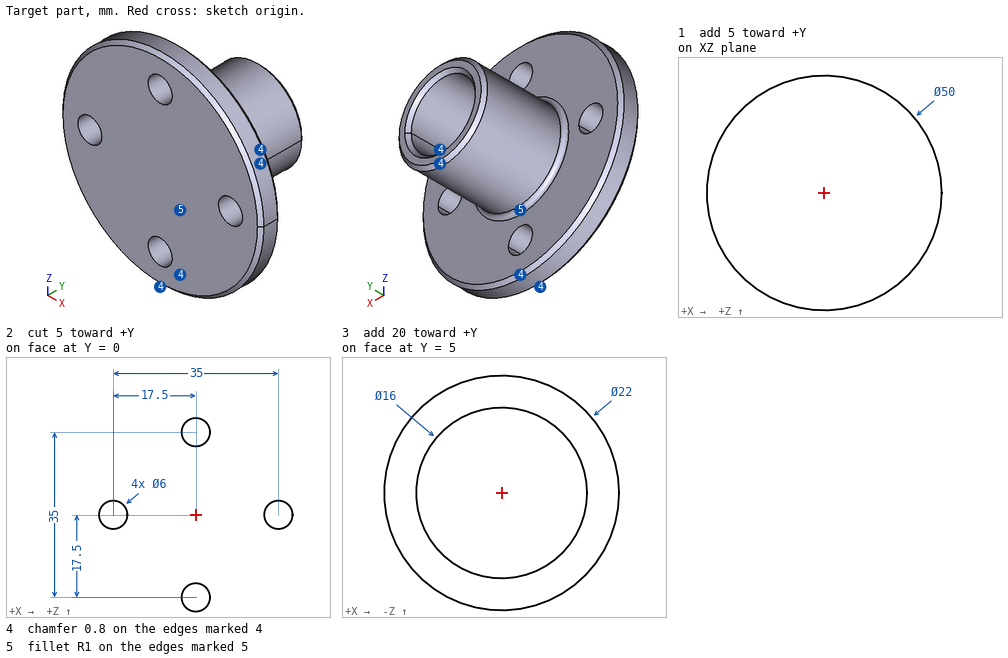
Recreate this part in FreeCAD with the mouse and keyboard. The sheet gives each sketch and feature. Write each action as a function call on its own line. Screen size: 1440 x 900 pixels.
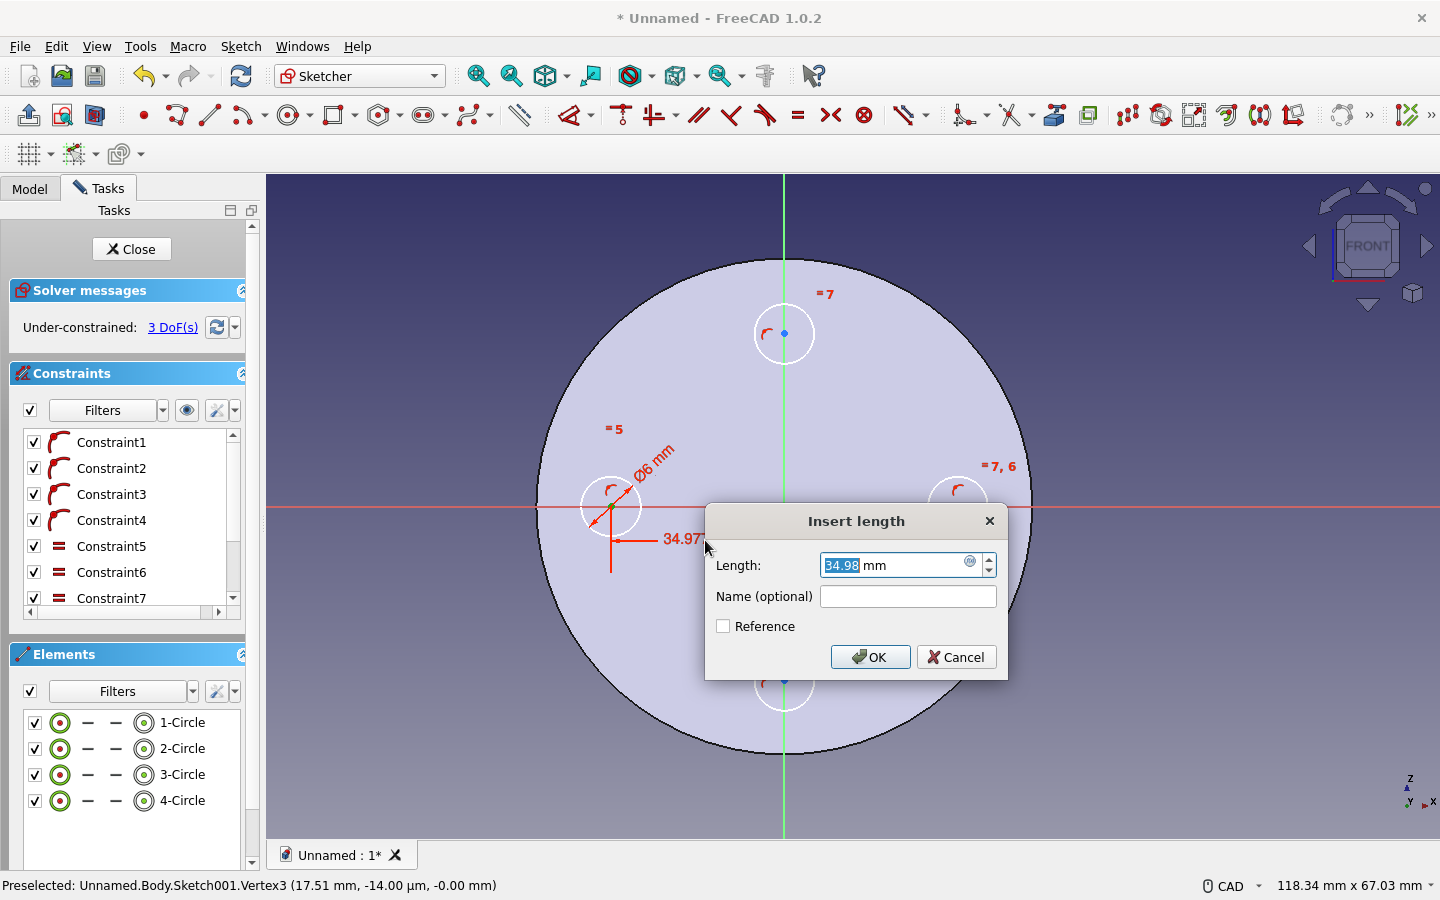
text(35)
key(Return)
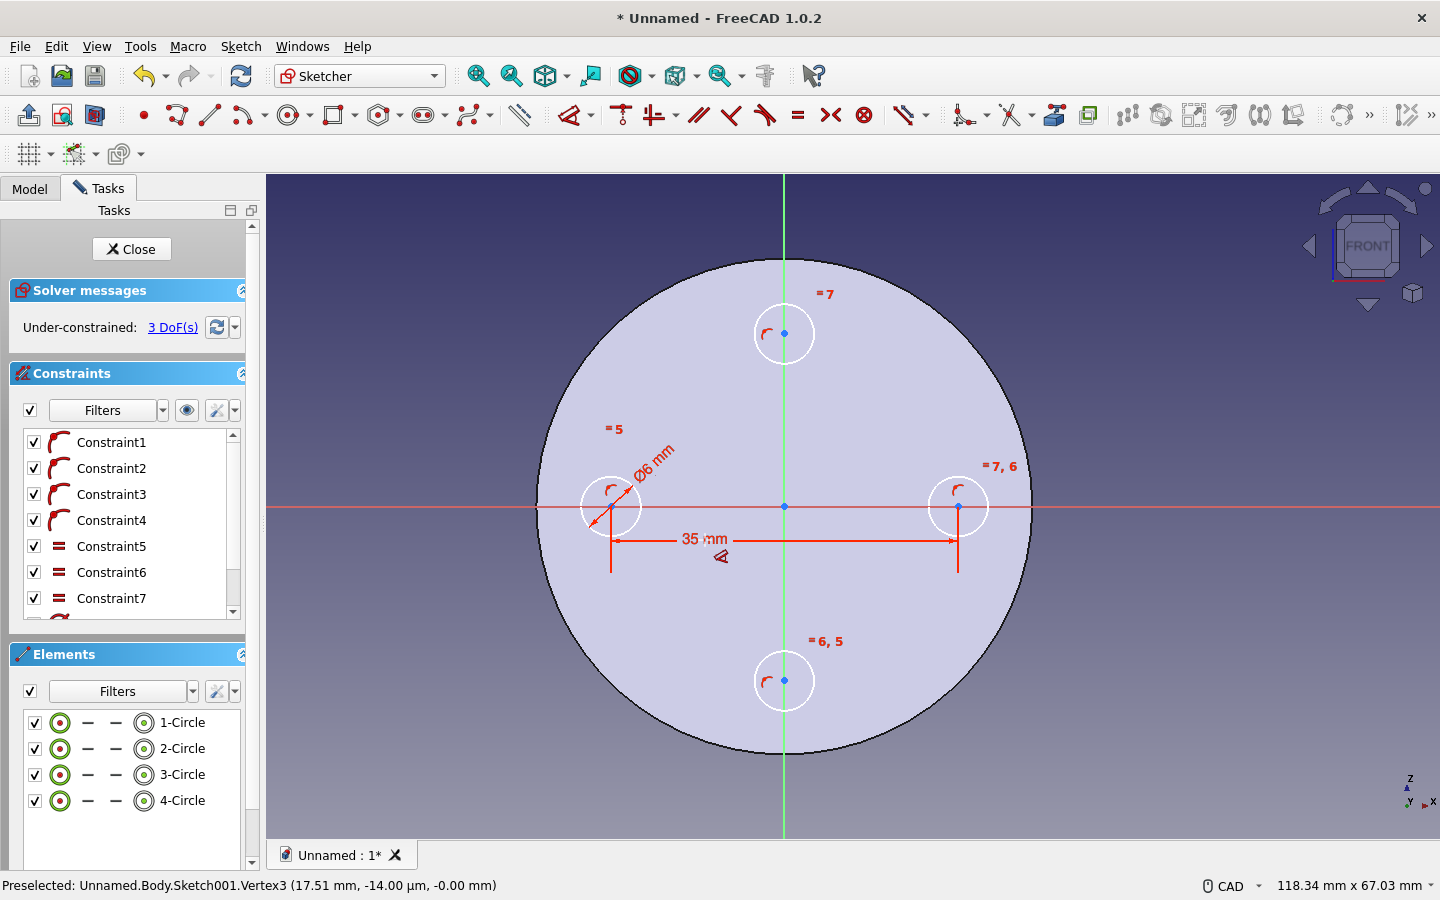
click(784, 681)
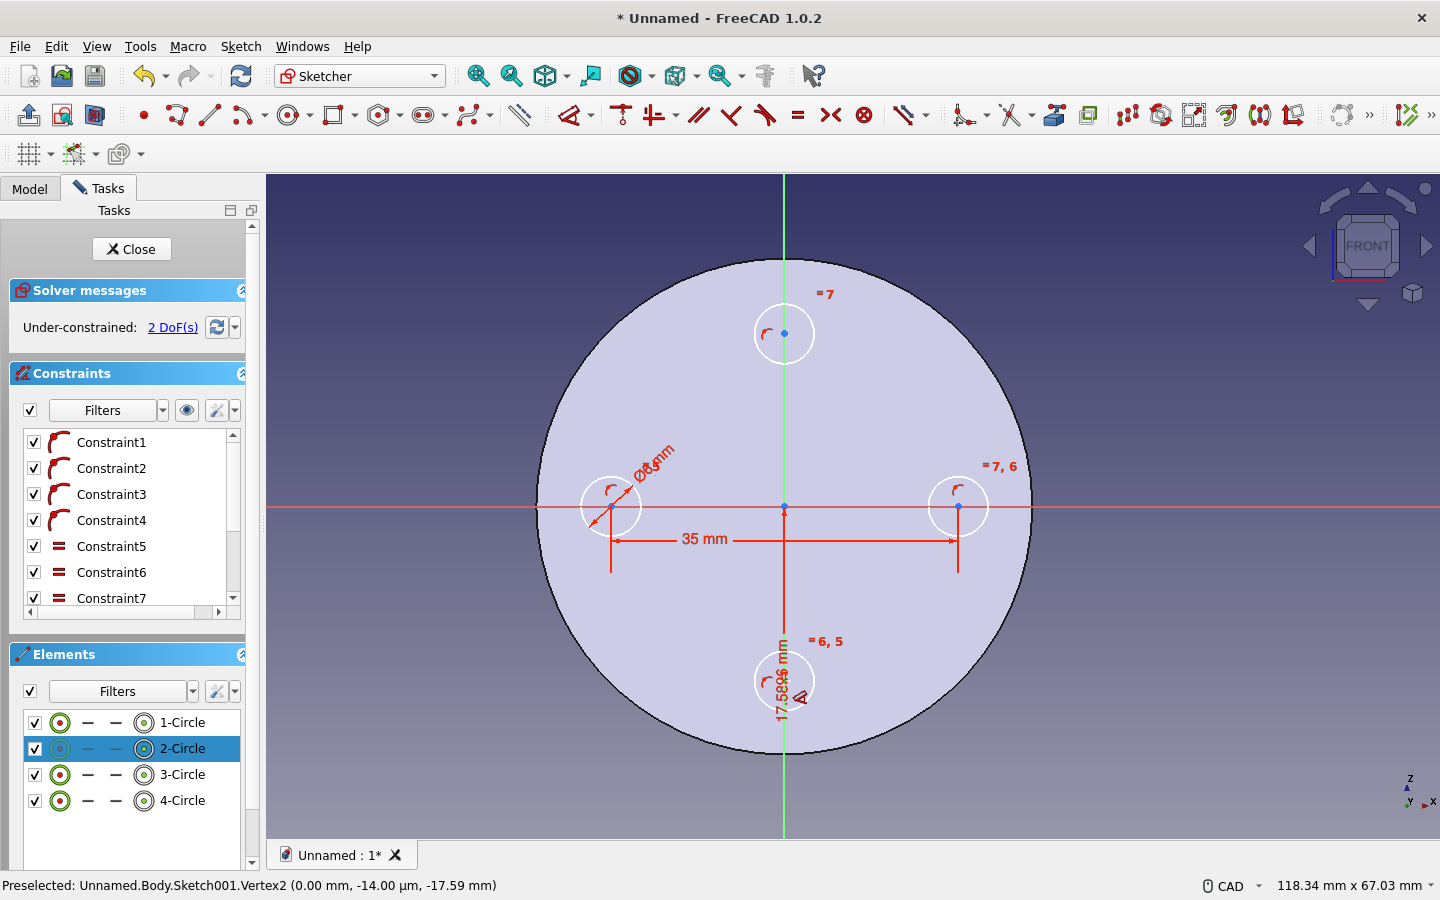
click(784, 334)
click(818, 428)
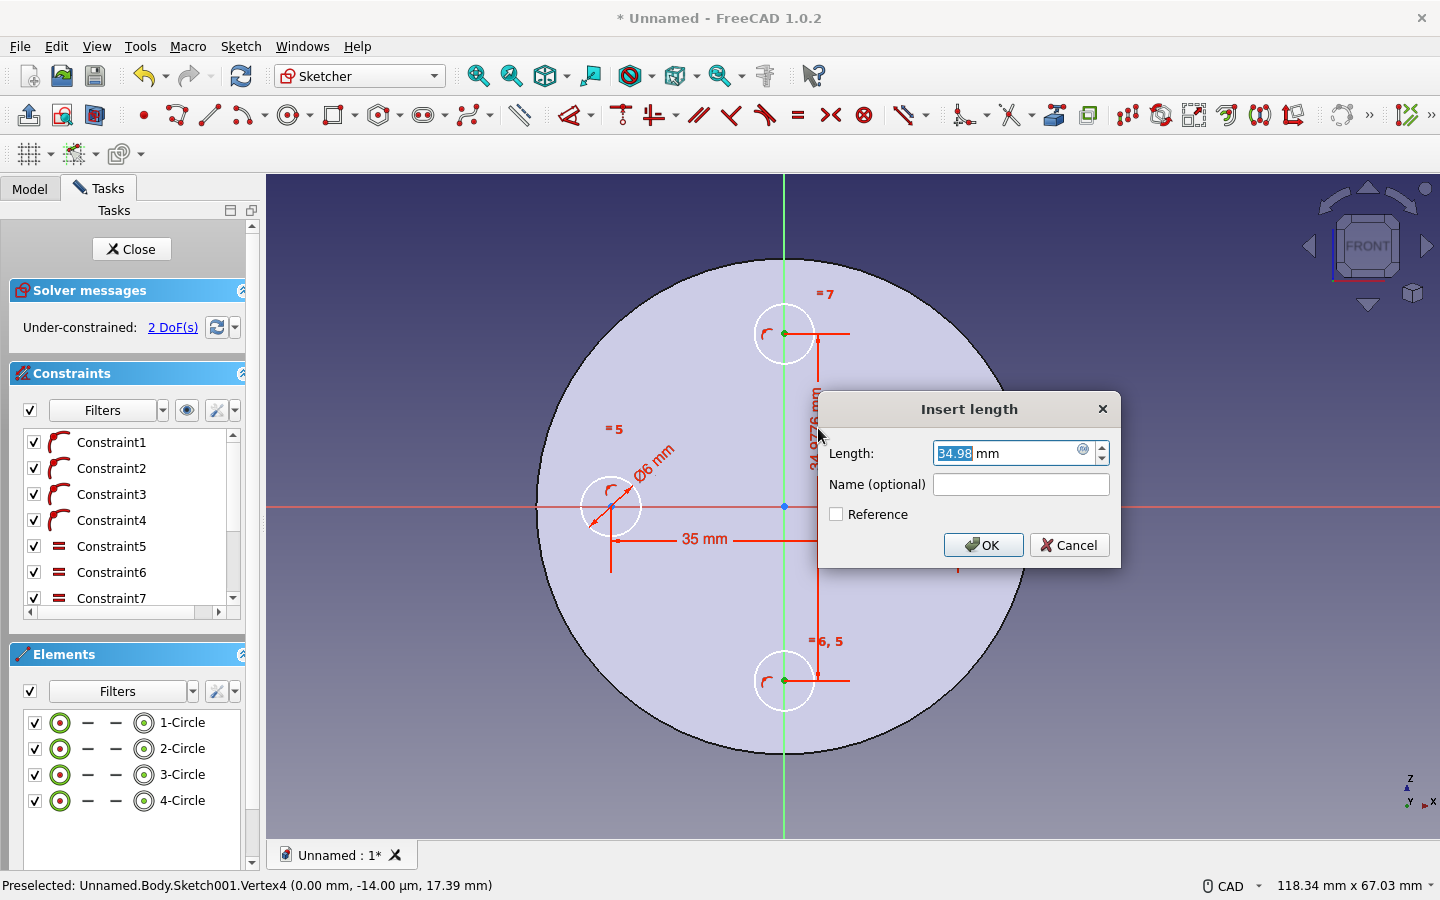
text(35)
key(Return)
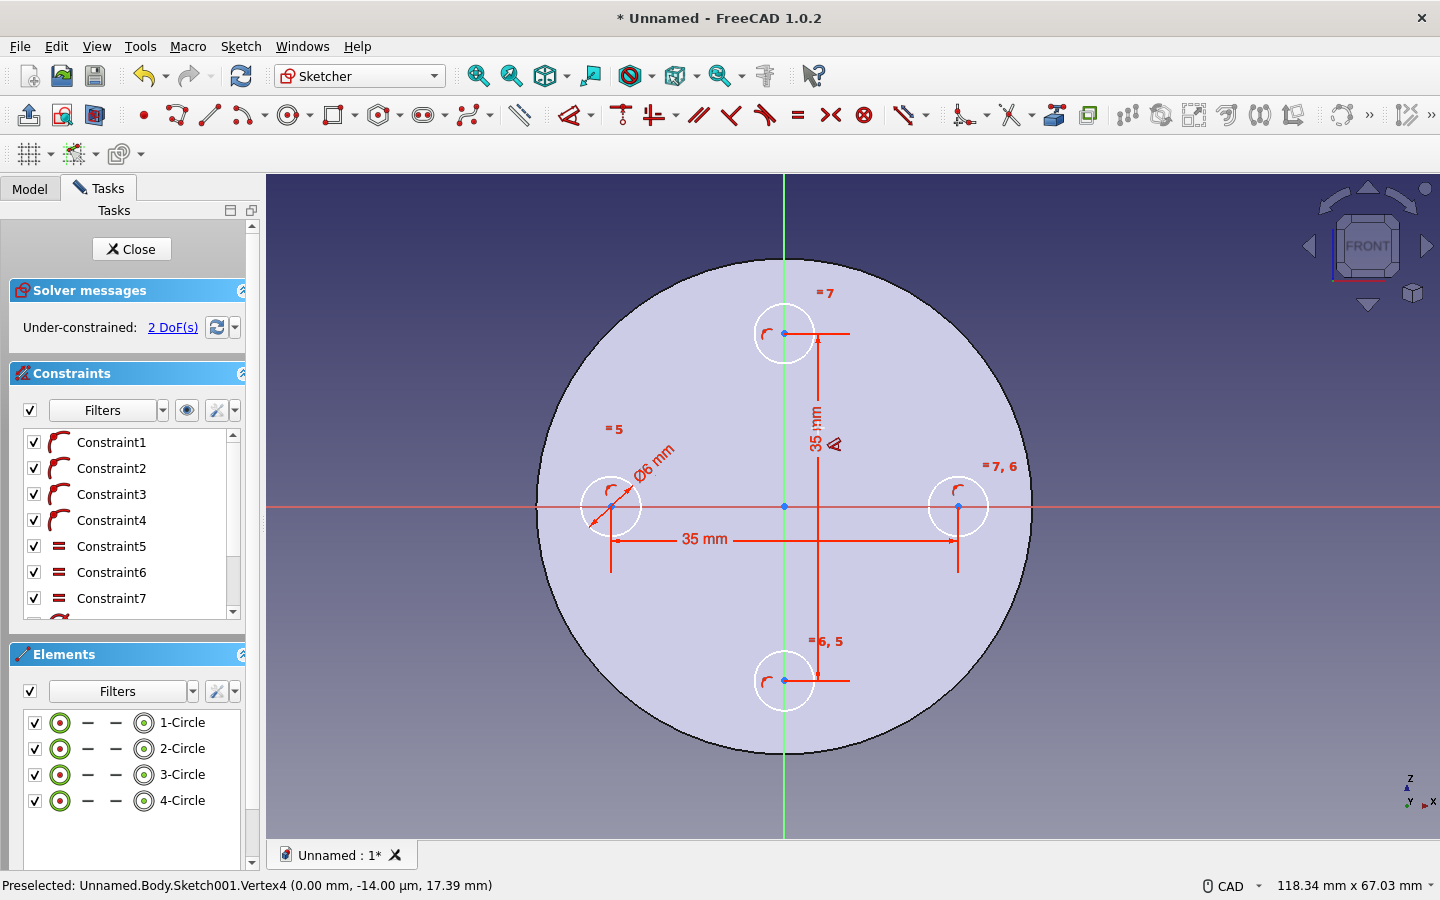
click(611, 506)
click(738, 472)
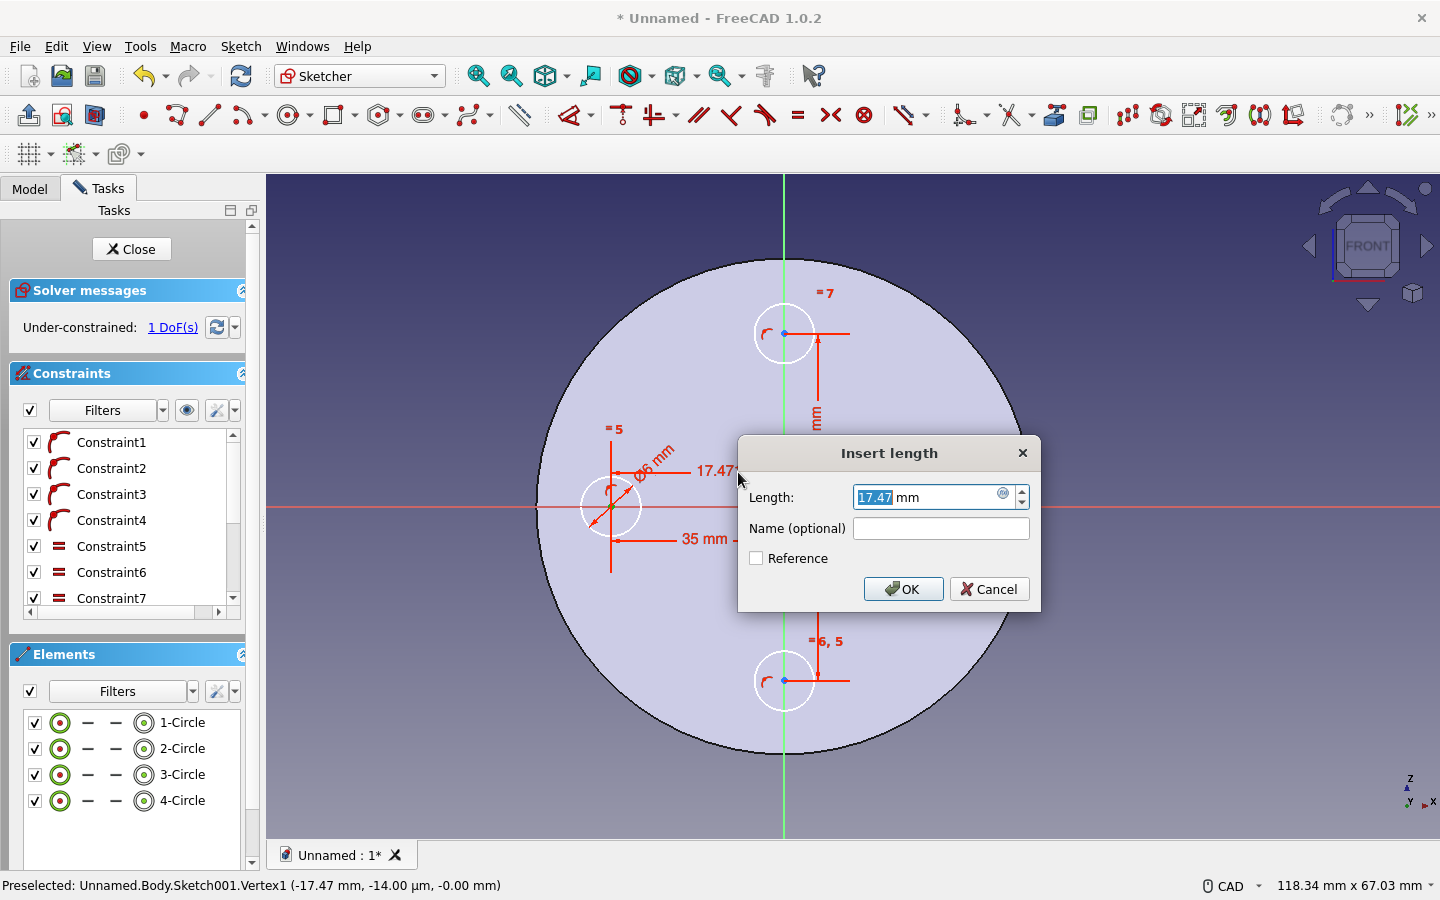
text(17.5)
key(Return)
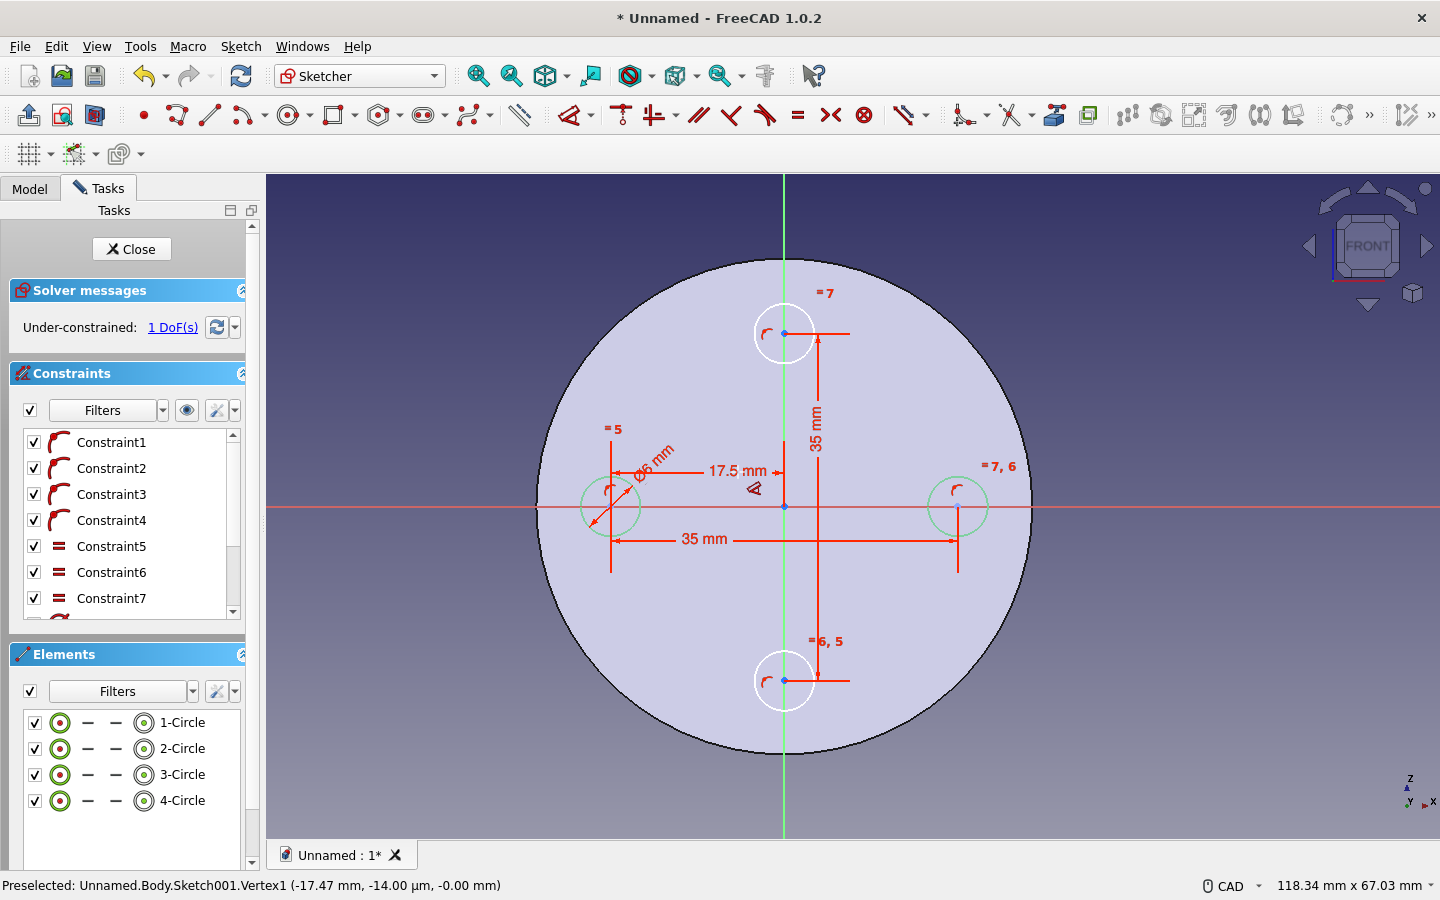
click(784, 681)
click(818, 594)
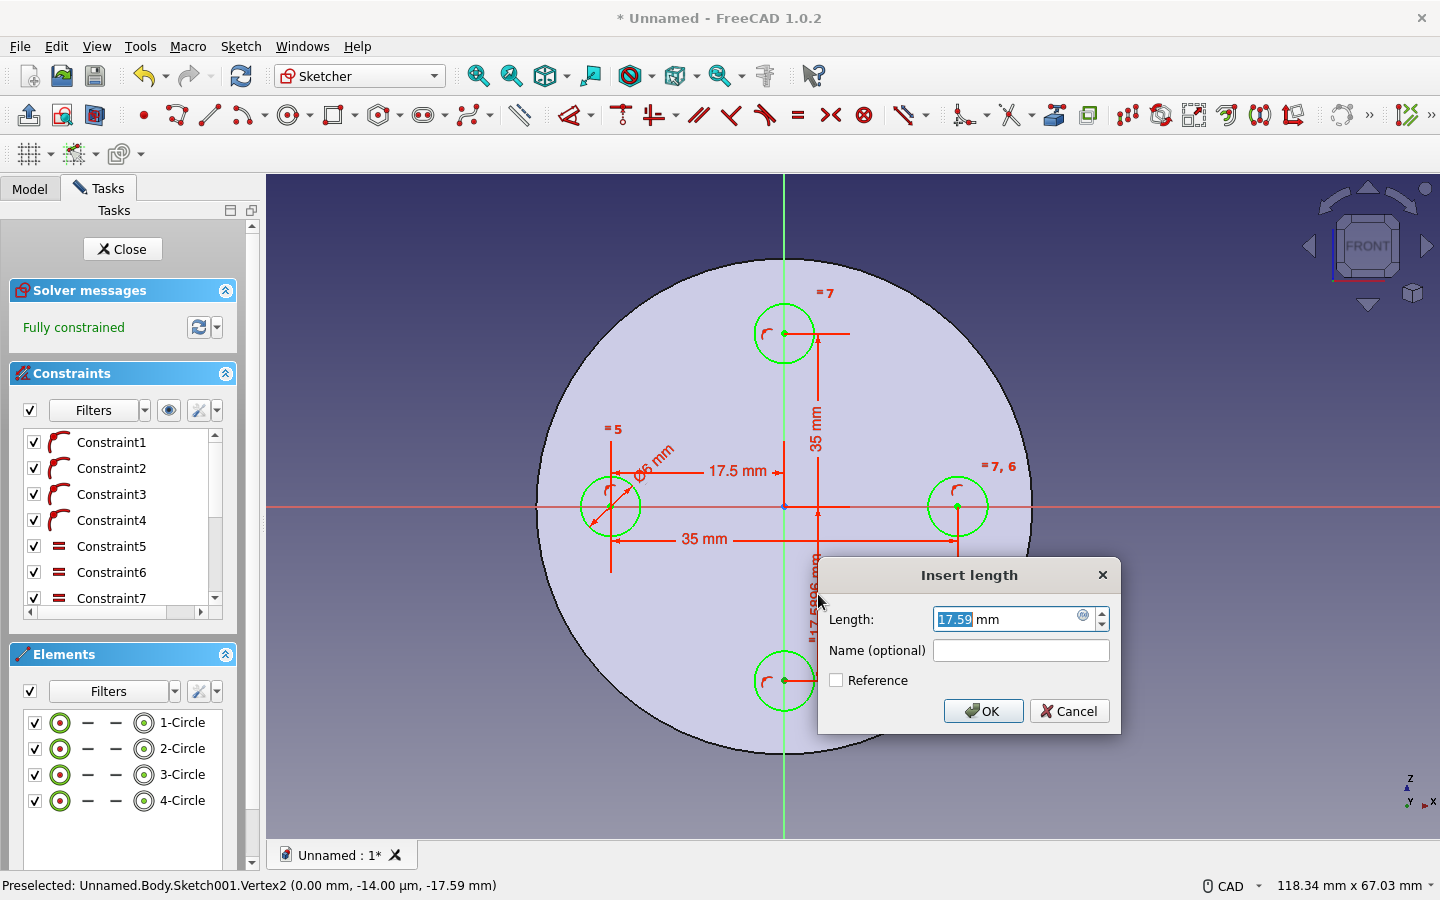
text(17.5)
key(Return)
key(Escape)